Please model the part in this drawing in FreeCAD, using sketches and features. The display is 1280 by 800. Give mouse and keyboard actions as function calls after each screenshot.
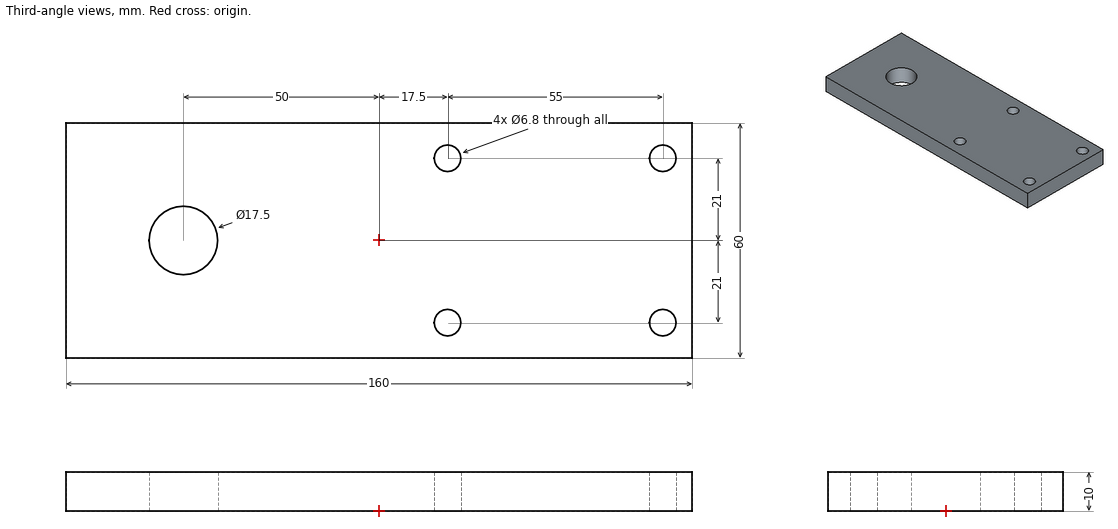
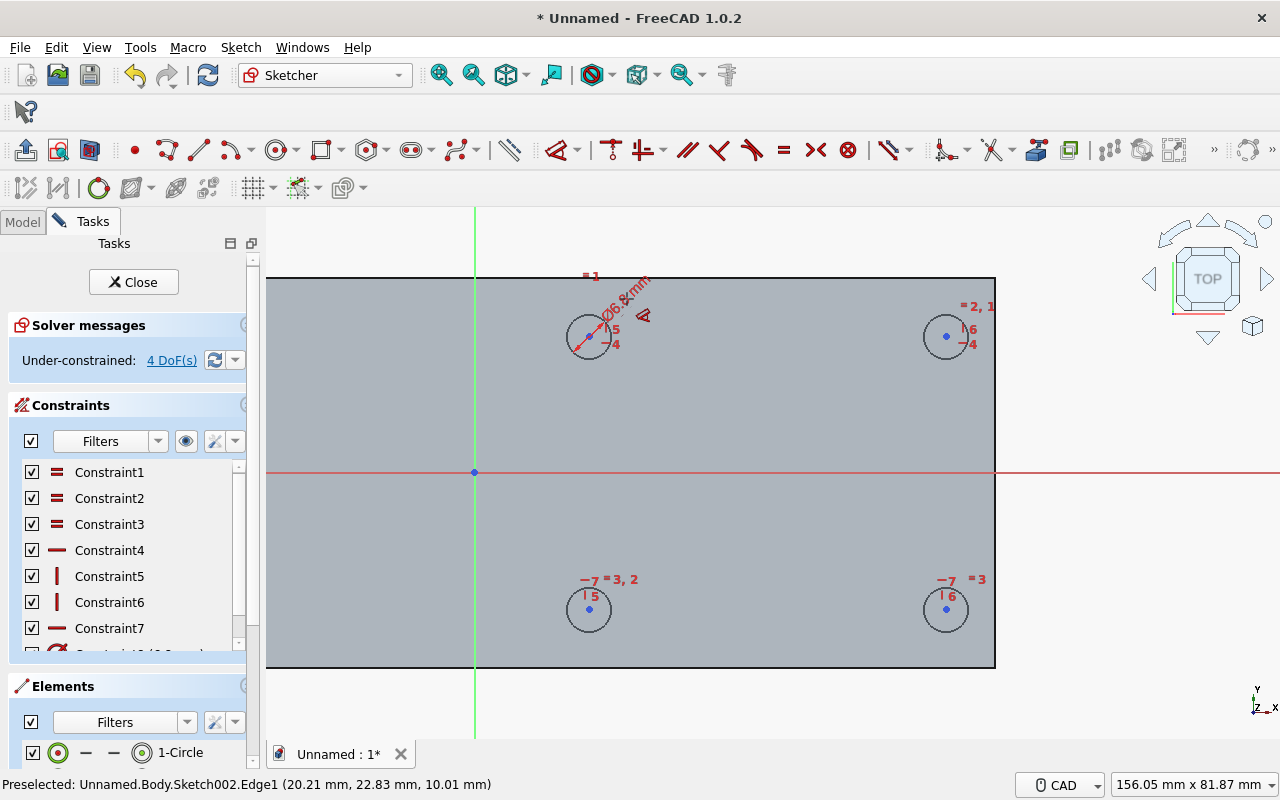
click(589, 337)
click(441, 405)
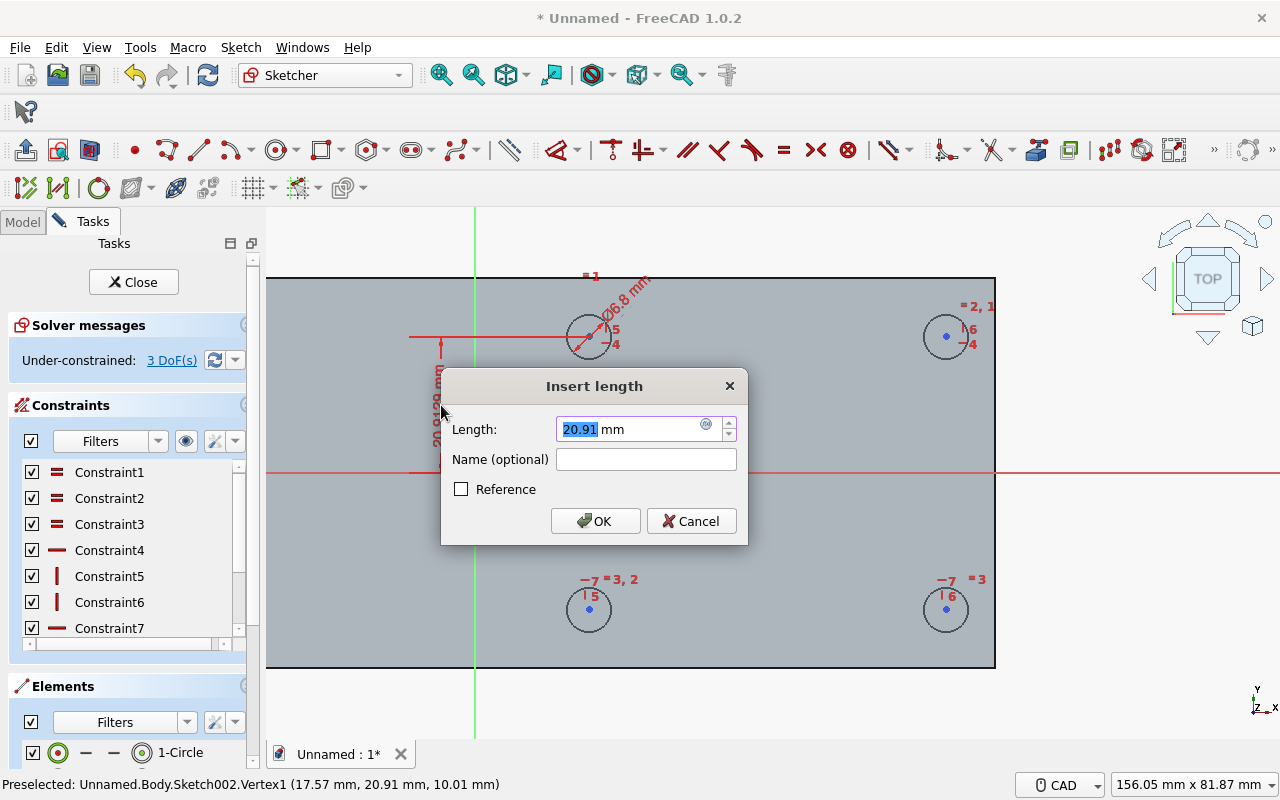
text(21)
key(Return)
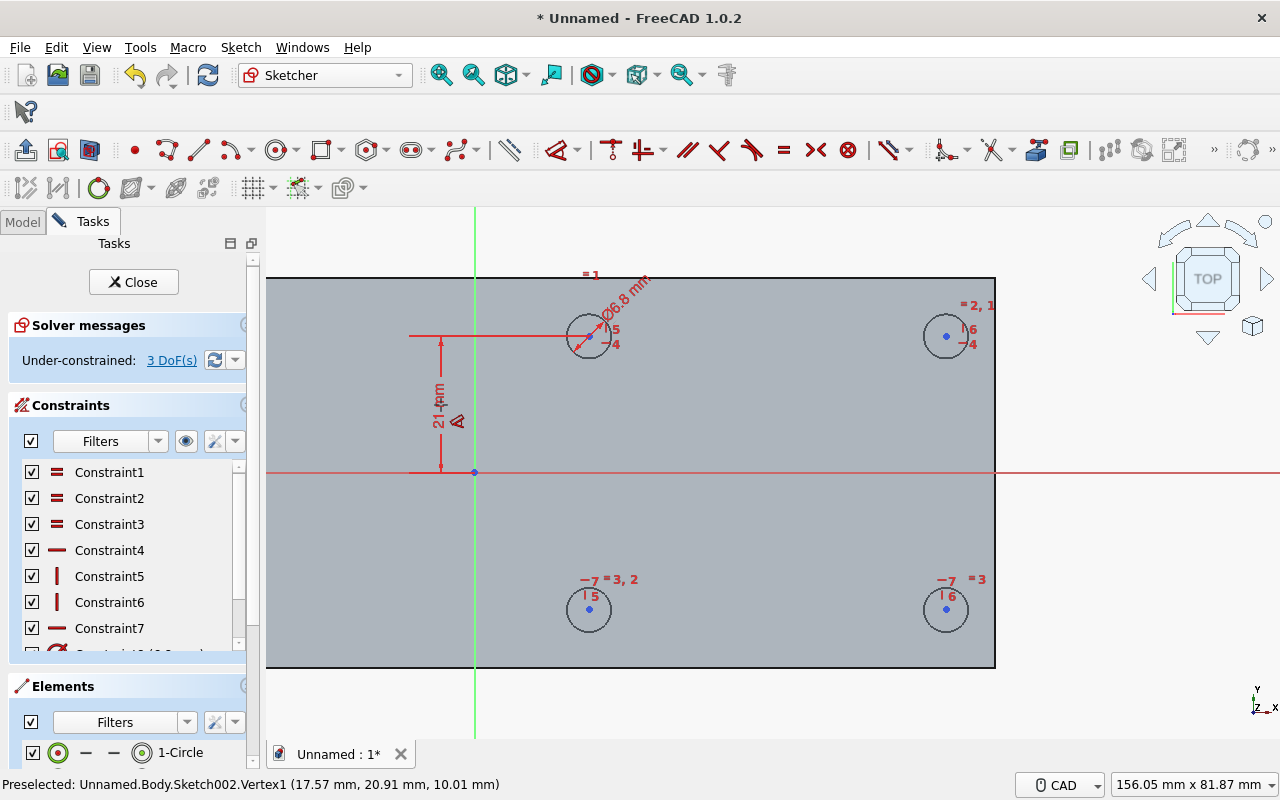
click(589, 610)
click(441, 541)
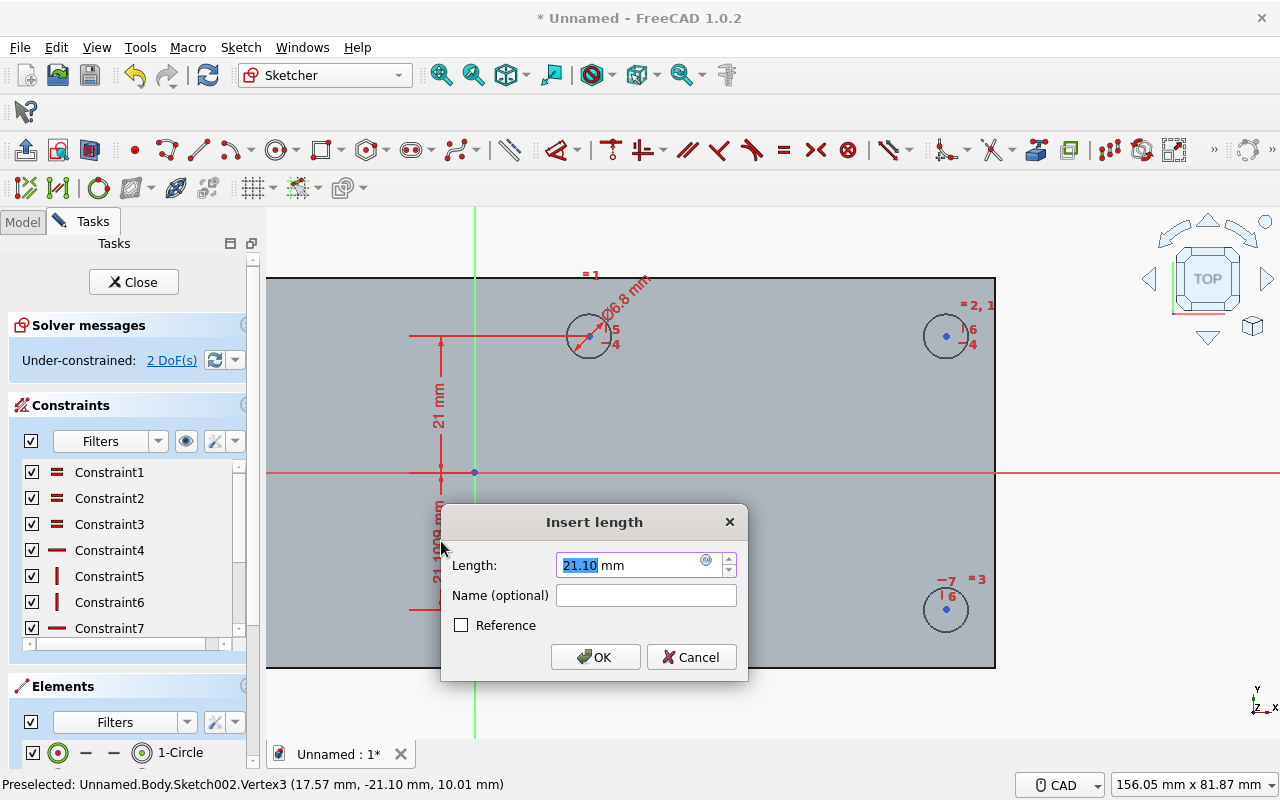
text(21)
key(Return)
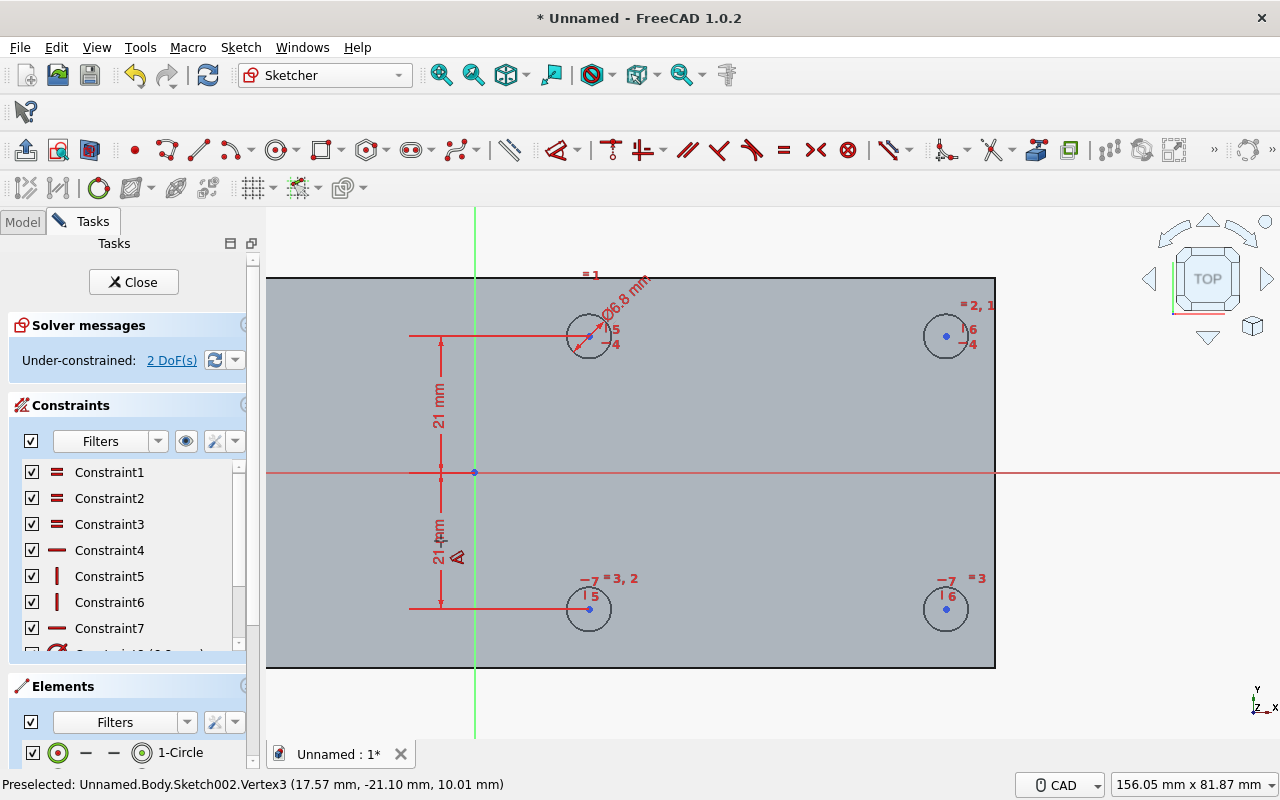
click(589, 336)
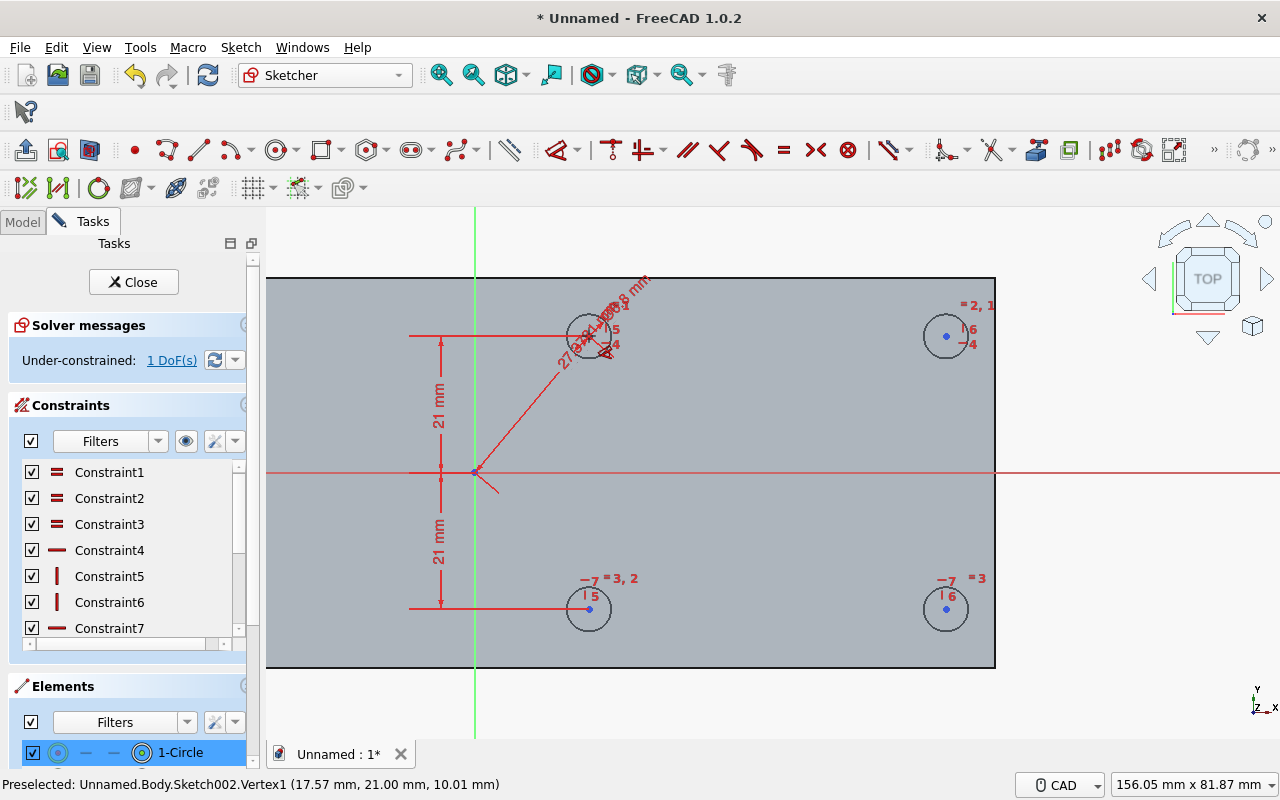
click(946, 336)
click(767, 302)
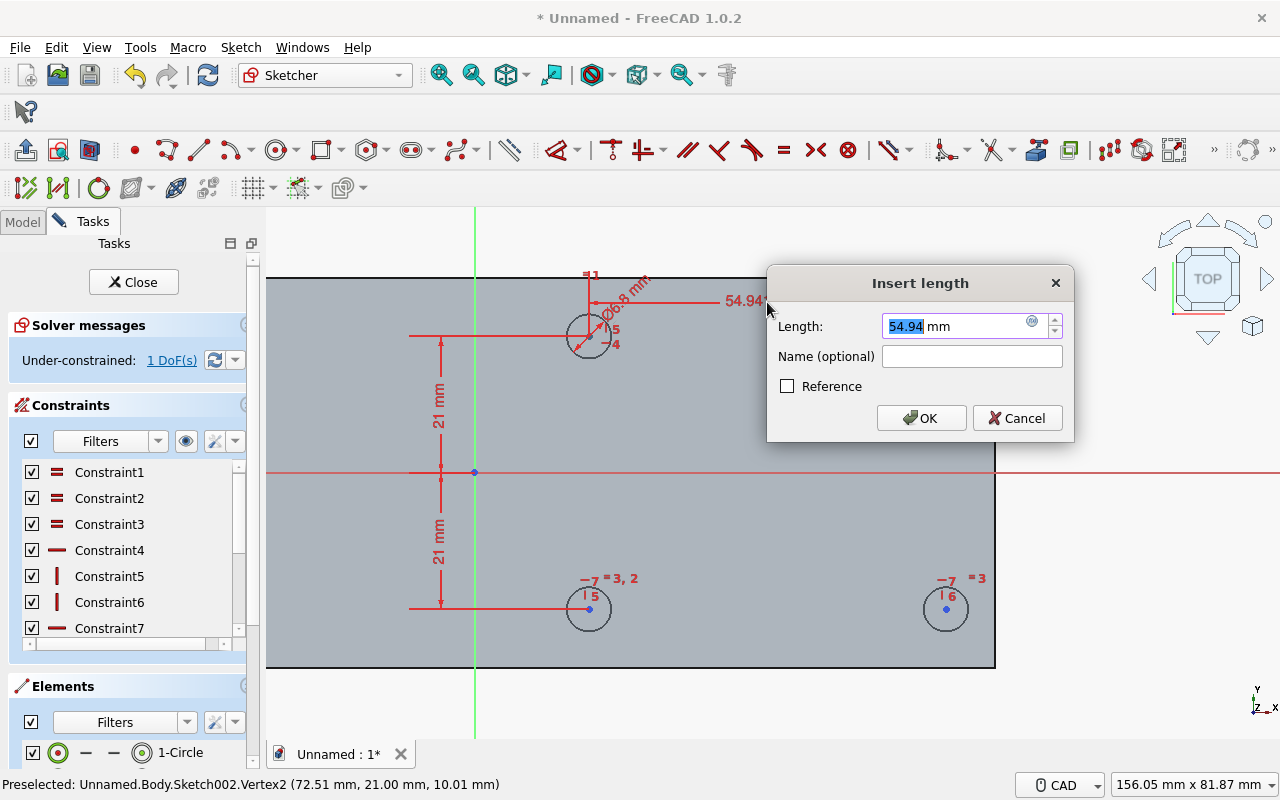
text(55)
key(Return)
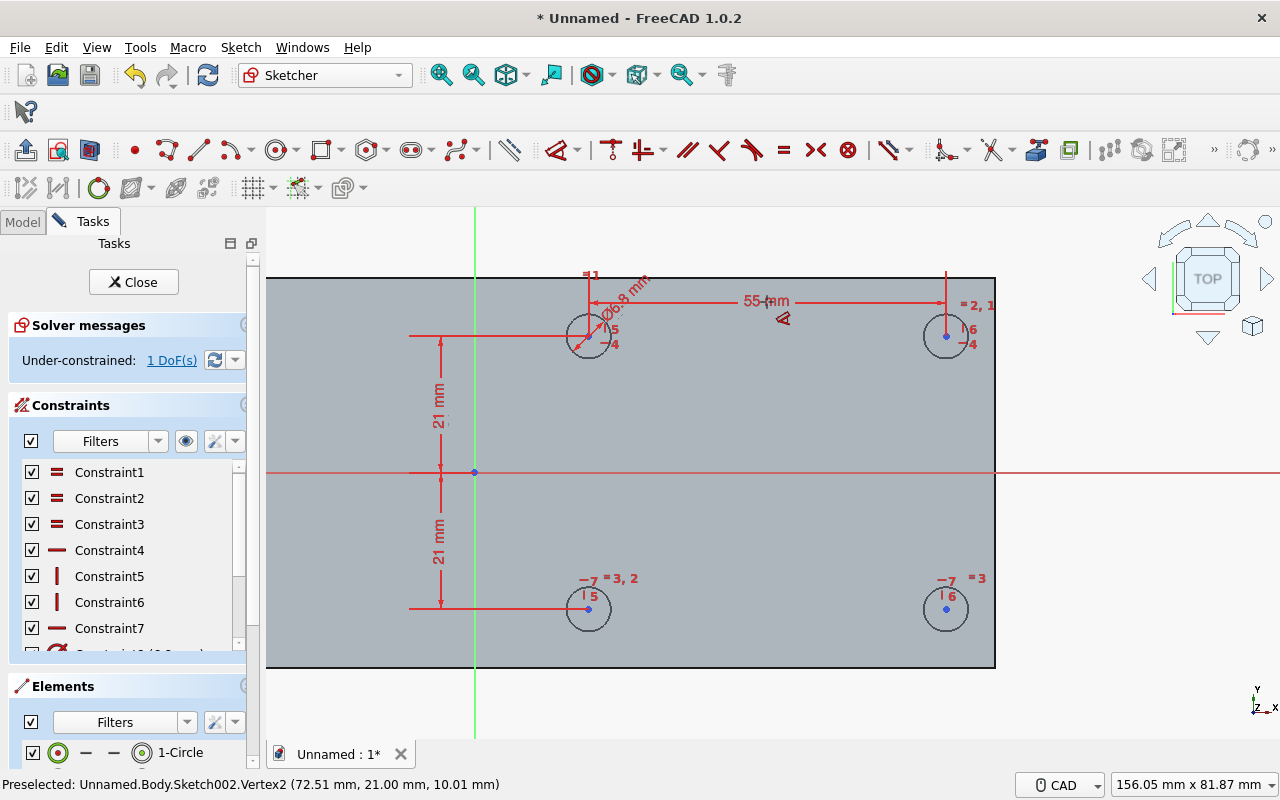
click(589, 336)
click(532, 302)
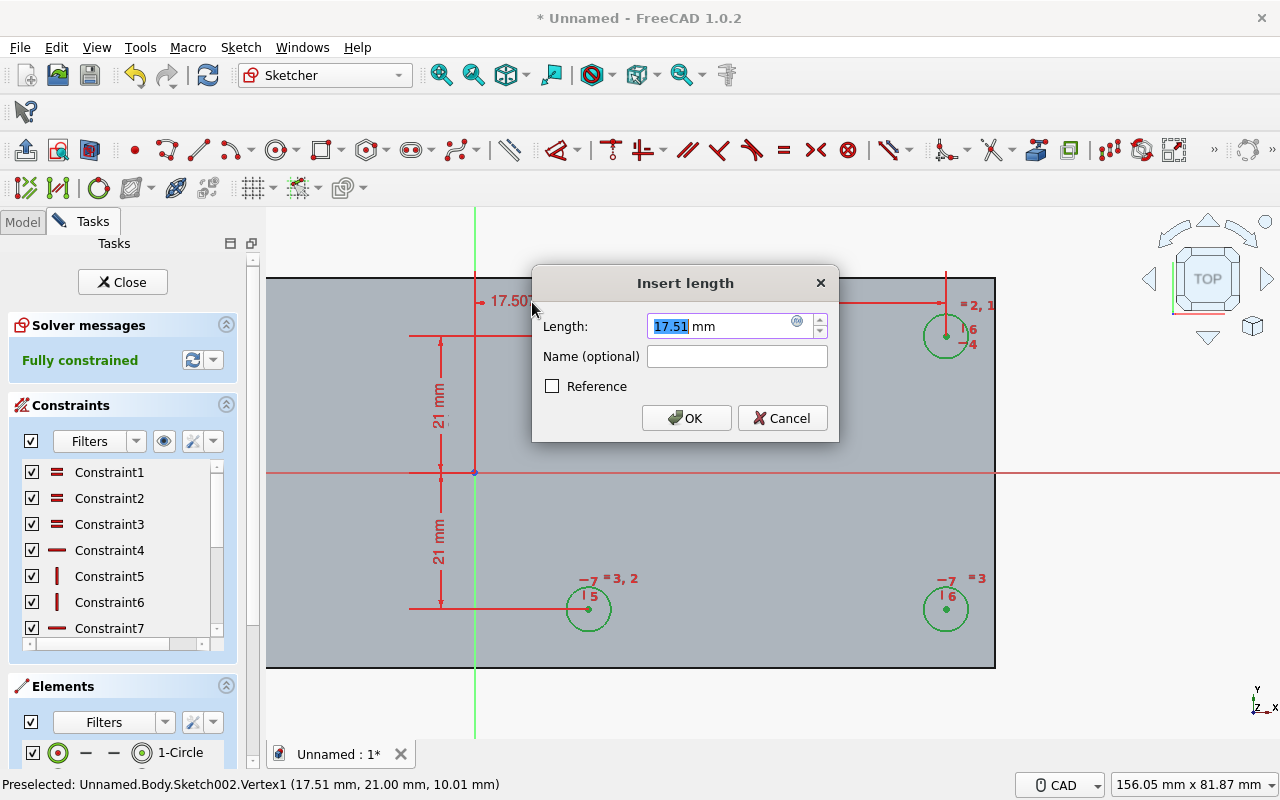
text(17.5)
key(Return)
key(Escape)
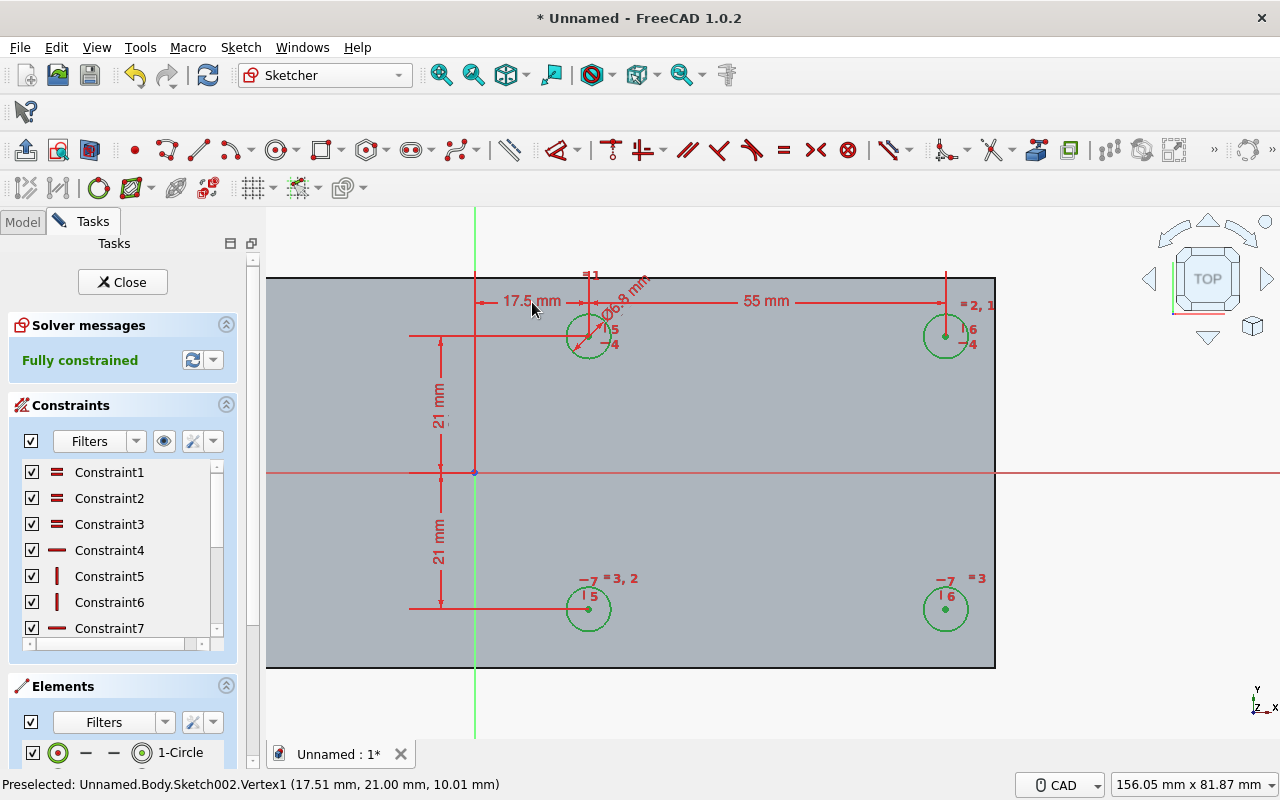
click(123, 282)